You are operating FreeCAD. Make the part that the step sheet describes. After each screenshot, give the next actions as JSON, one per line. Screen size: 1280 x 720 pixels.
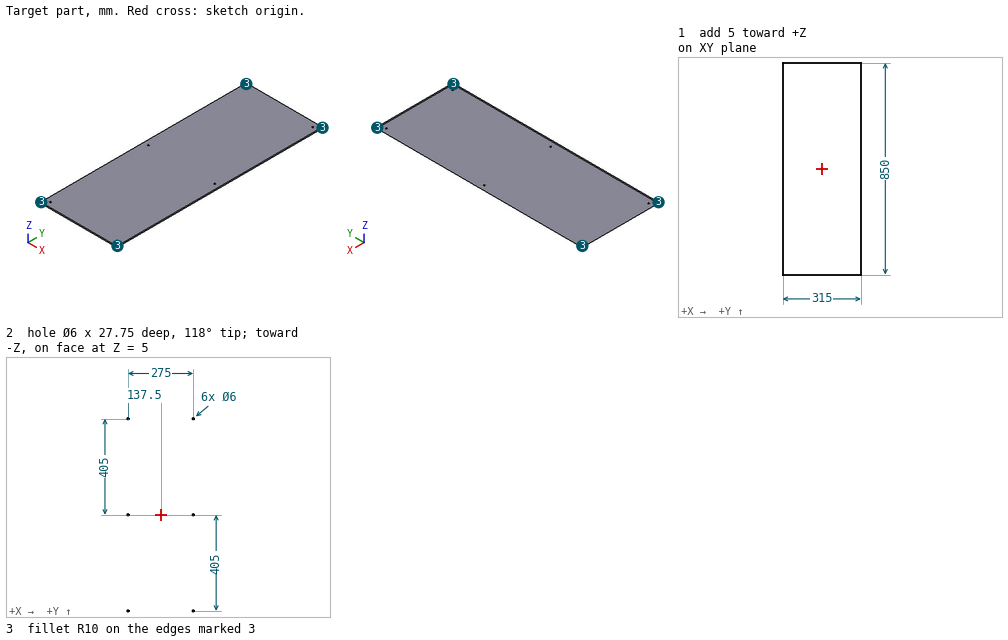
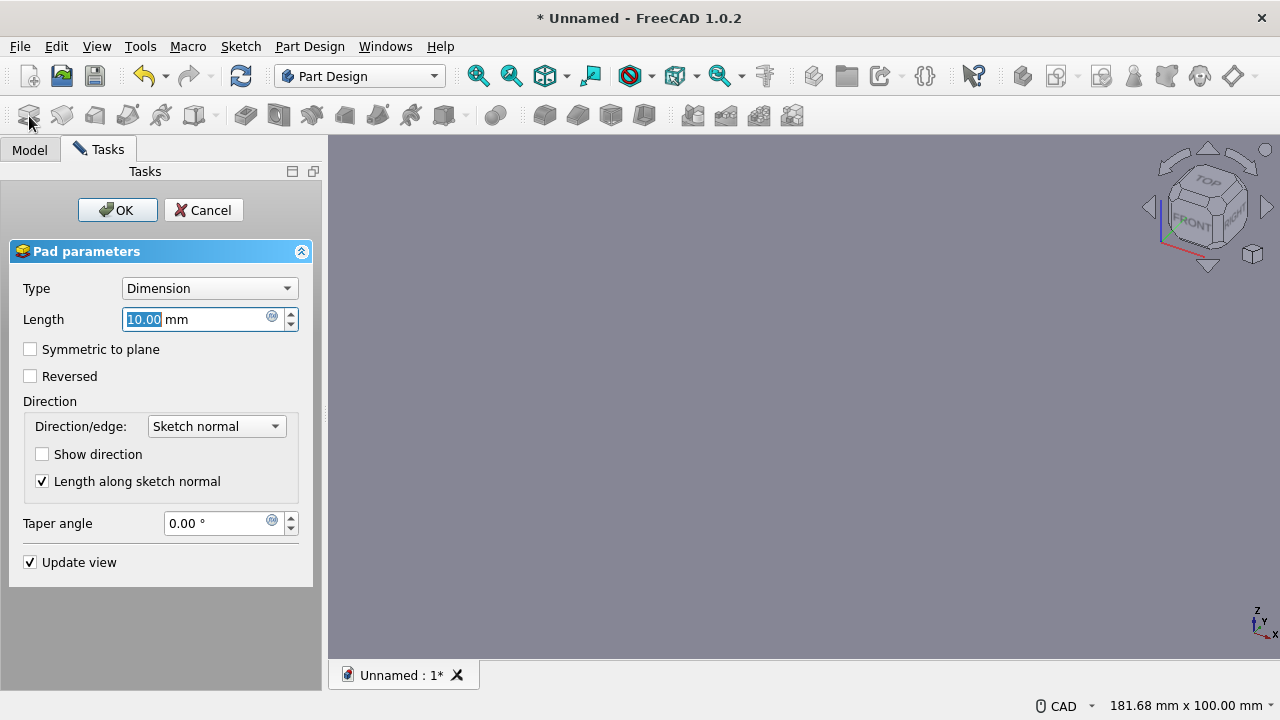
{"action": "type", "text": "5"}
{"action": "key", "text": "Tab"}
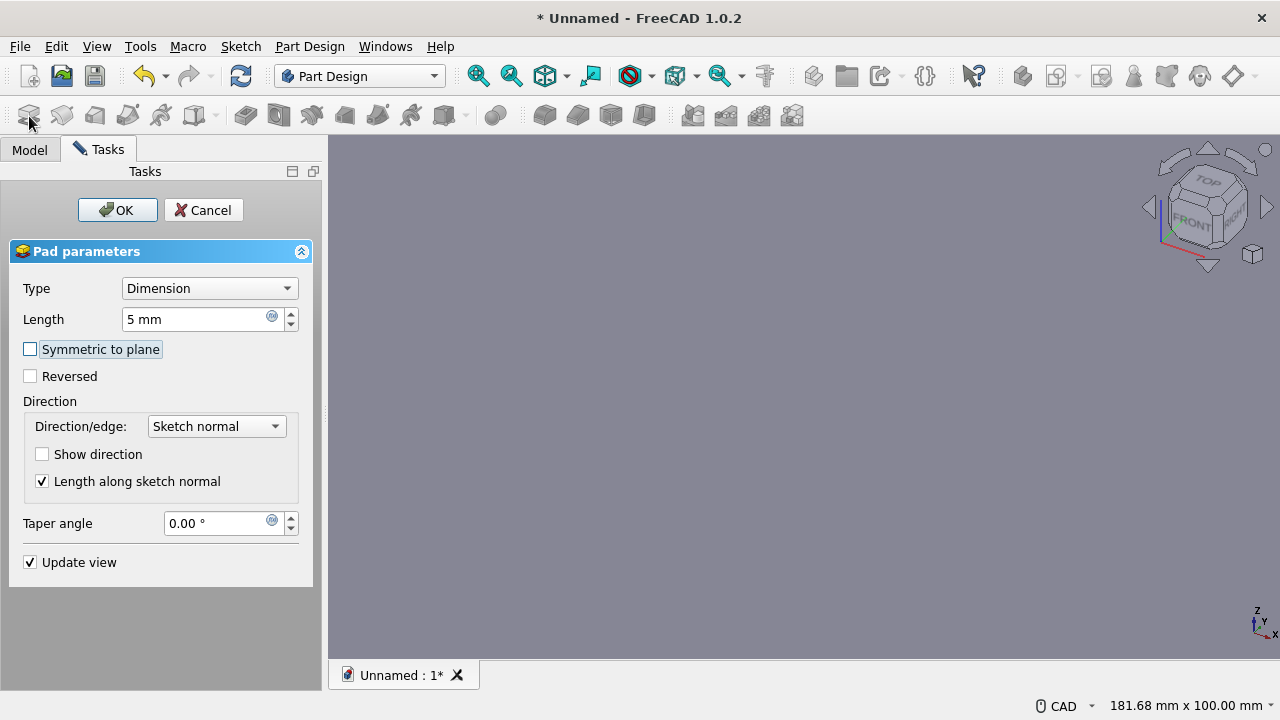
{"action": "left_click", "coordinate": [118, 210]}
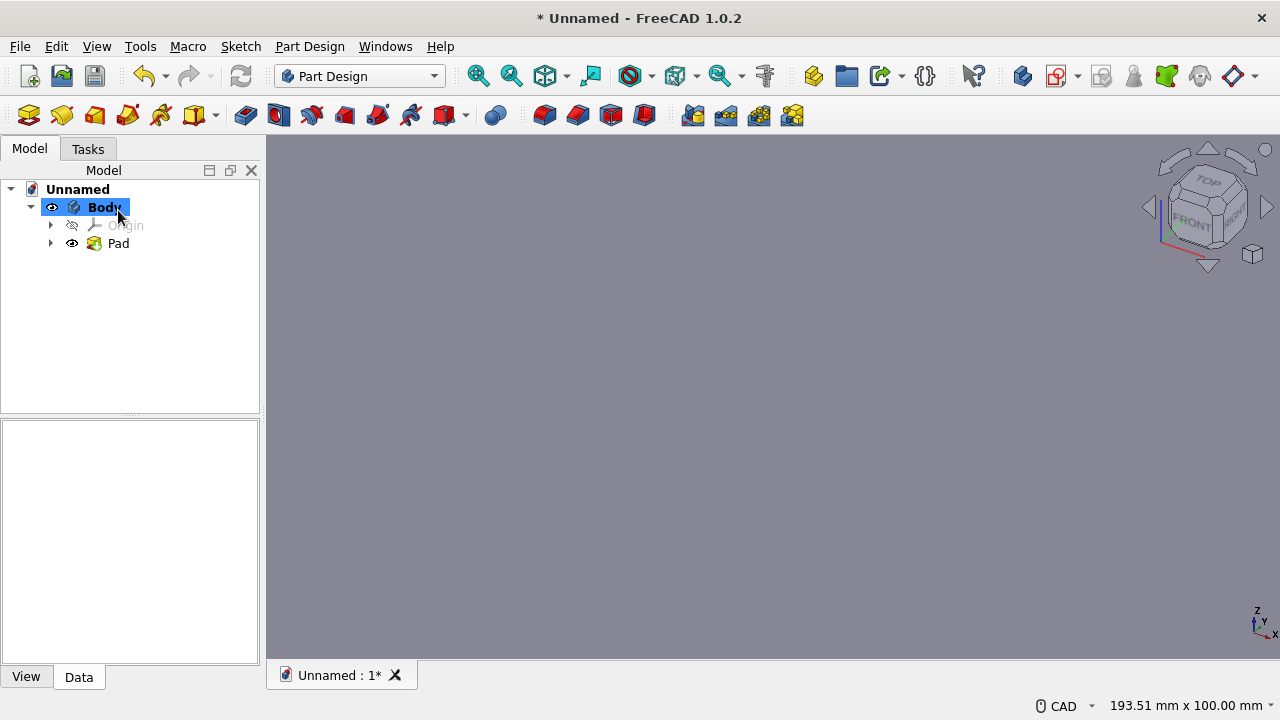
{"action": "key", "text": "v f"}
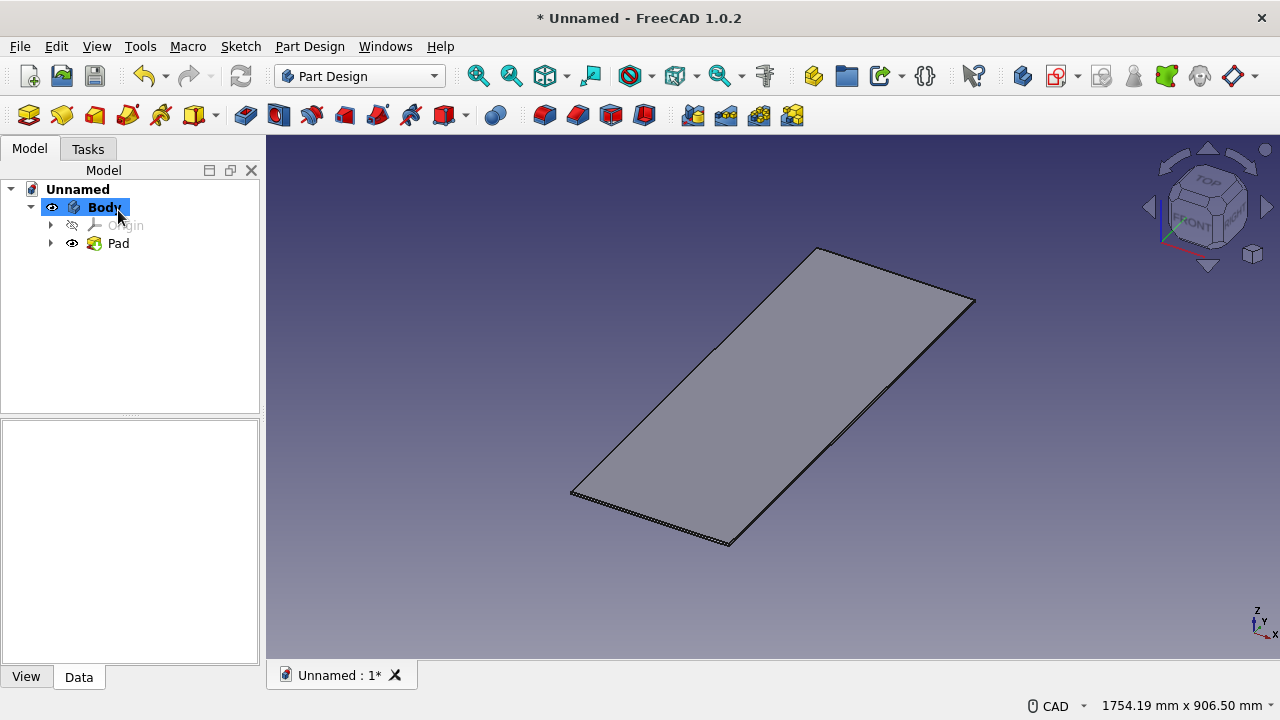
{"action": "left_click", "coordinate": [843, 325]}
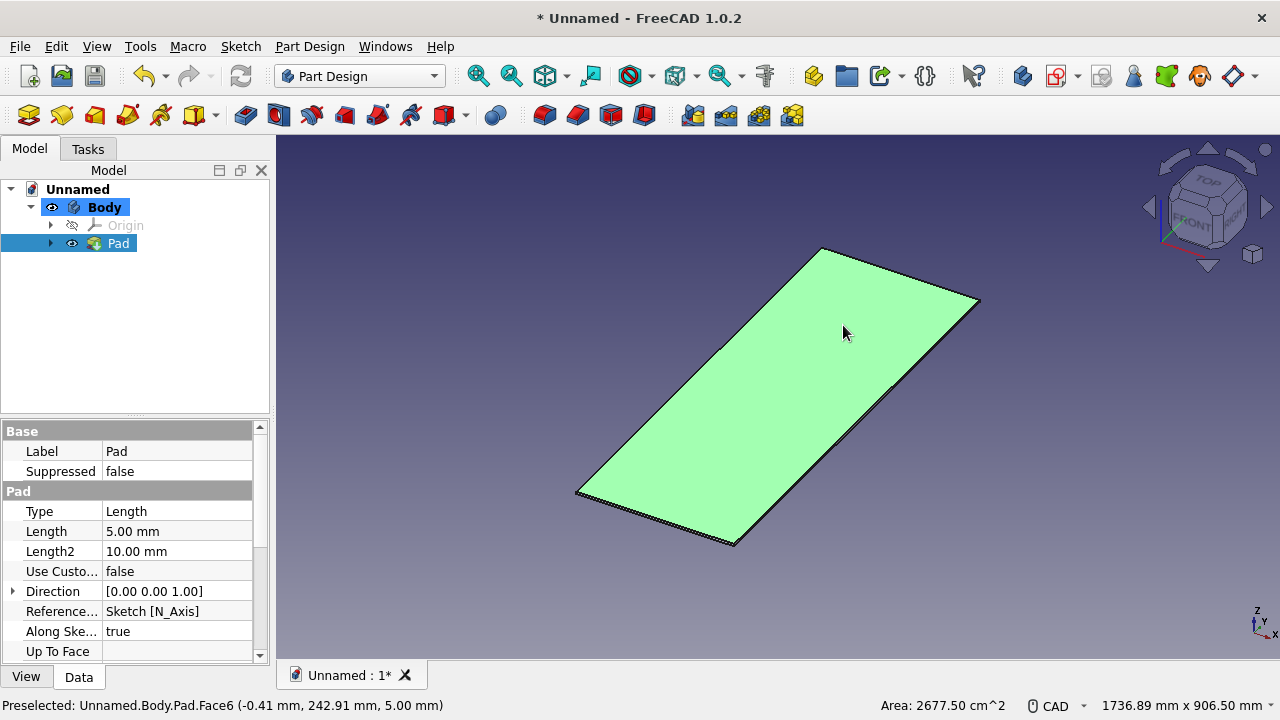
{"action": "left_click", "coordinate": [1056, 76]}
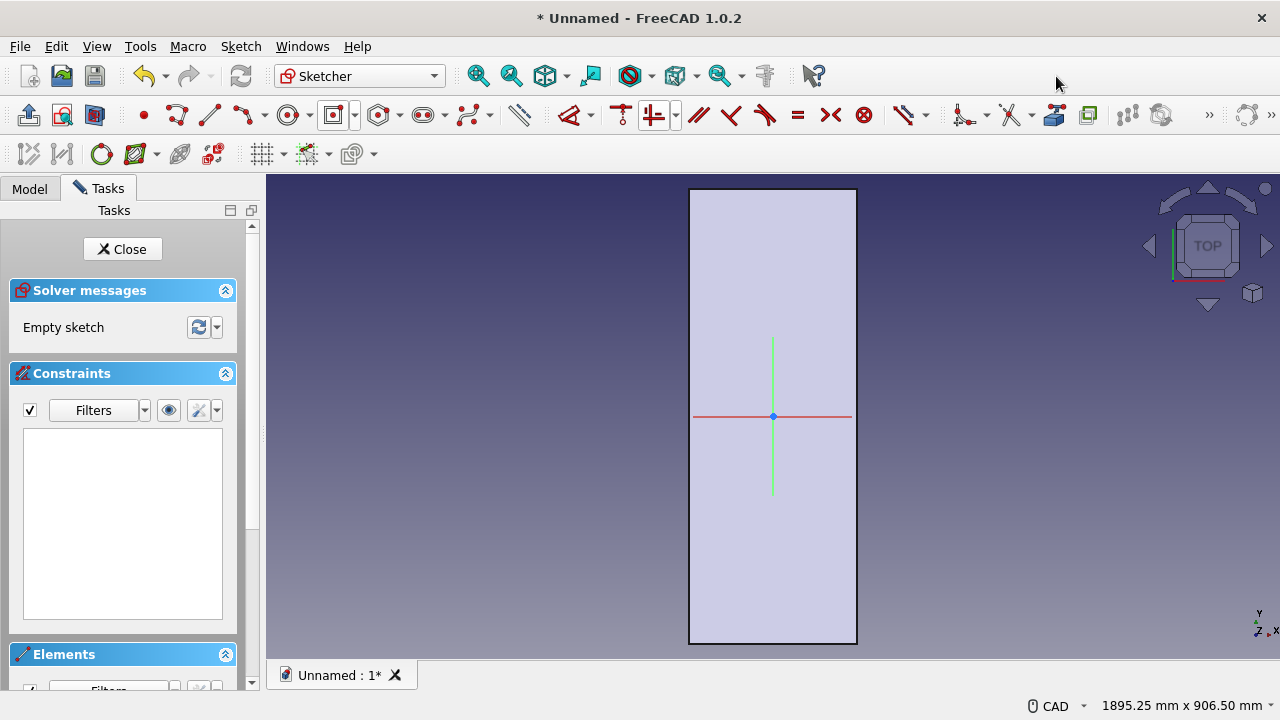
{"action": "scroll", "coordinate": [565, 416], "scroll_direction": "down", "scroll_amount": 2}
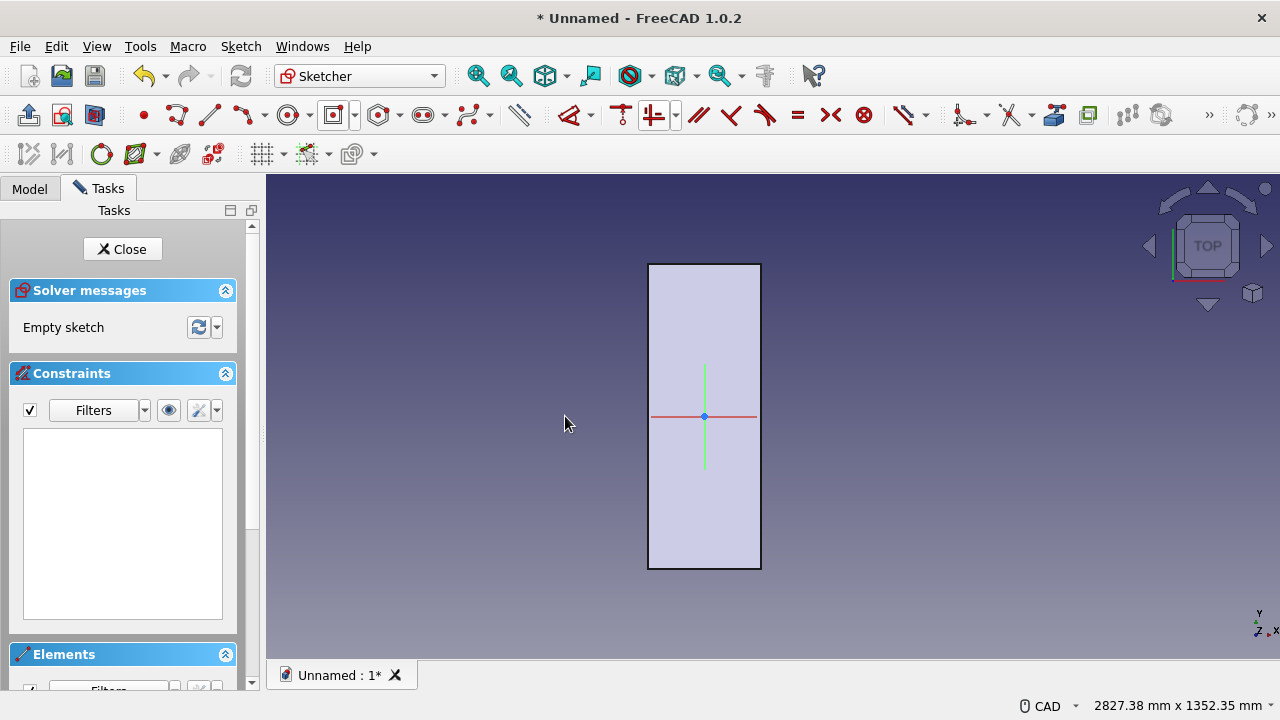
{"action": "key", "text": "g c"}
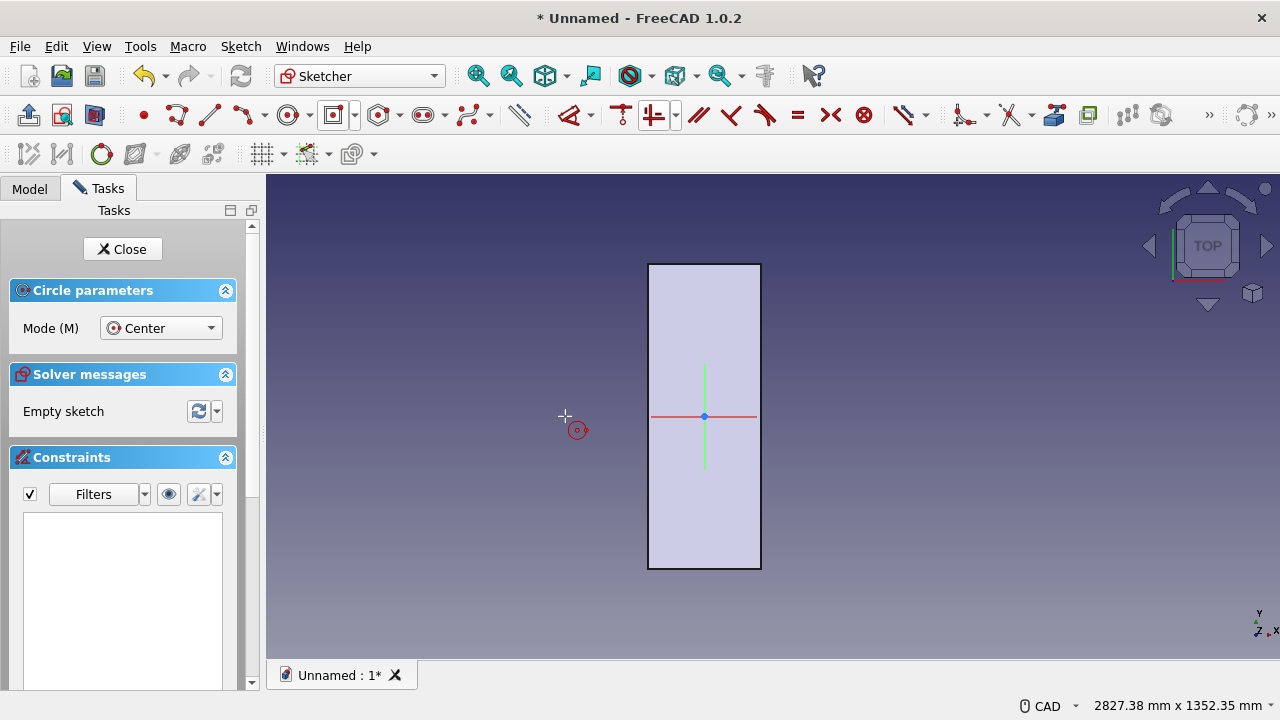
{"action": "scroll", "coordinate": [655, 271], "scroll_direction": "up", "scroll_amount": 16}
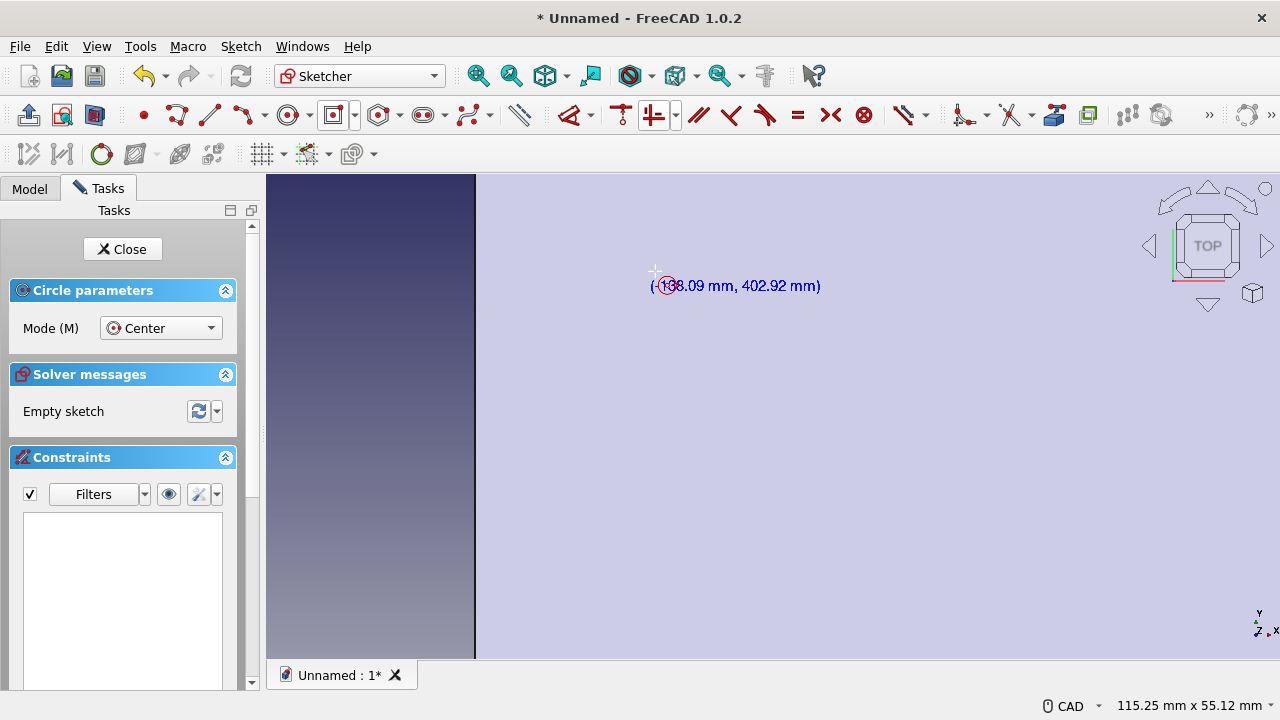
{"action": "scroll", "coordinate": [644, 237], "scroll_direction": "down", "scroll_amount": 15}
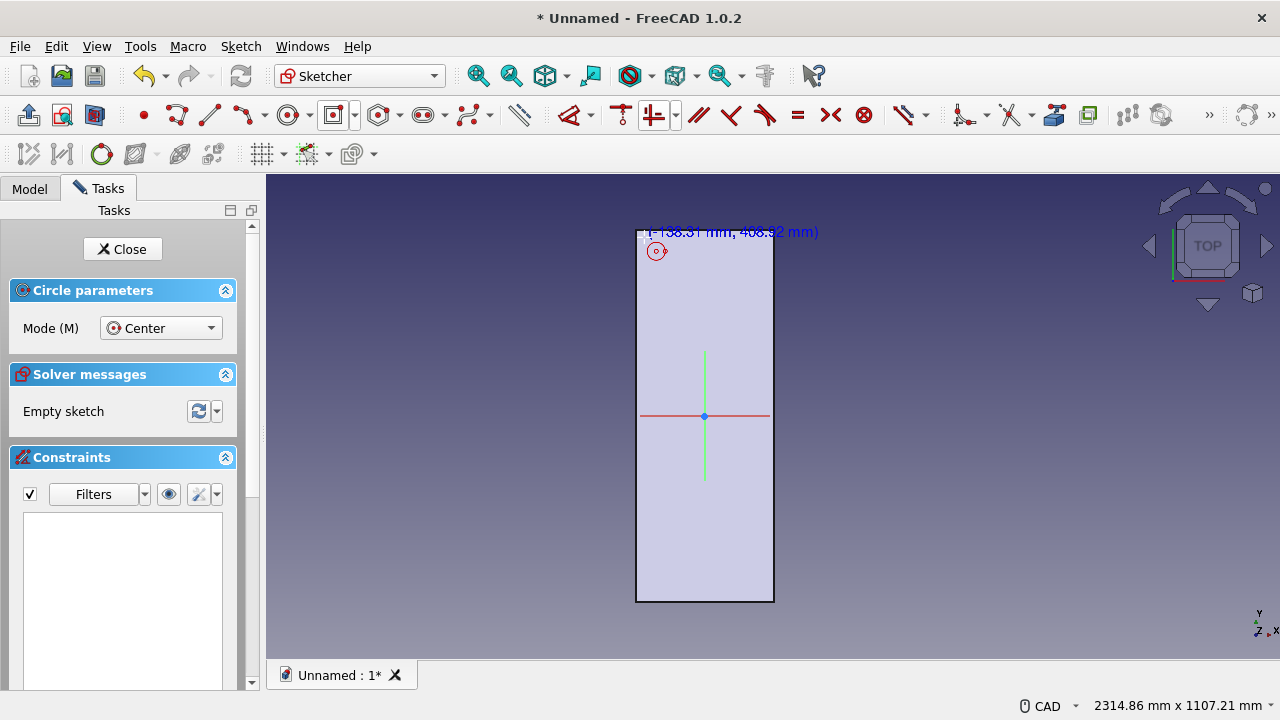
{"action": "left_click", "coordinate": [645, 239]}
{"action": "mouse_move", "coordinate": [646, 238]}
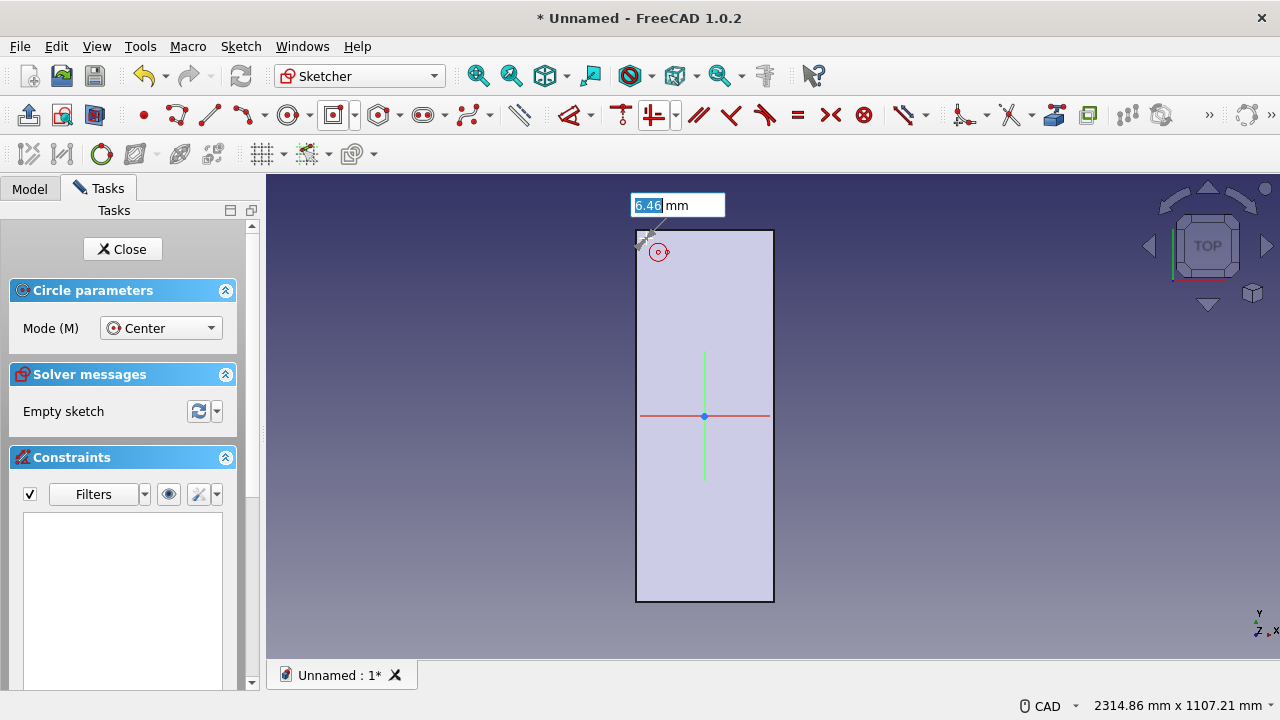
{"action": "type", "text": "6"}
{"action": "key", "text": "Return"}